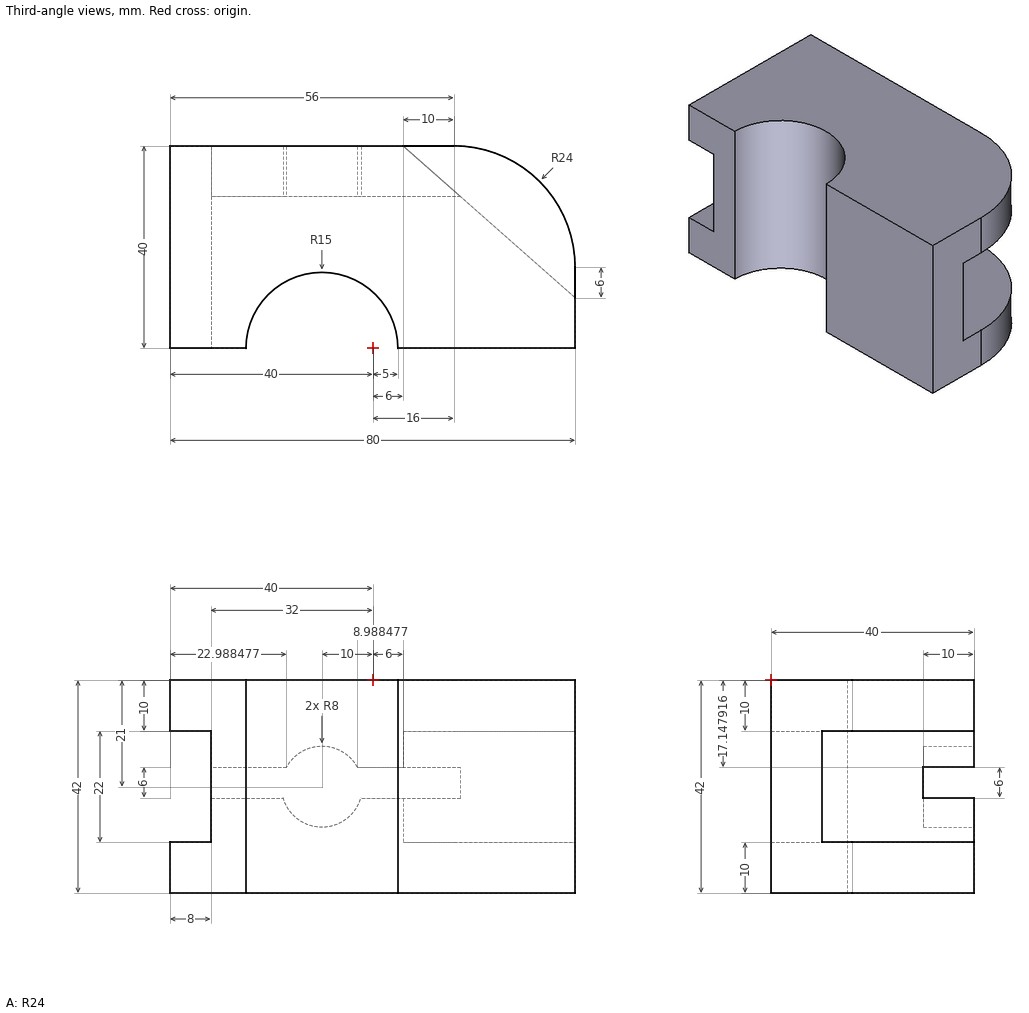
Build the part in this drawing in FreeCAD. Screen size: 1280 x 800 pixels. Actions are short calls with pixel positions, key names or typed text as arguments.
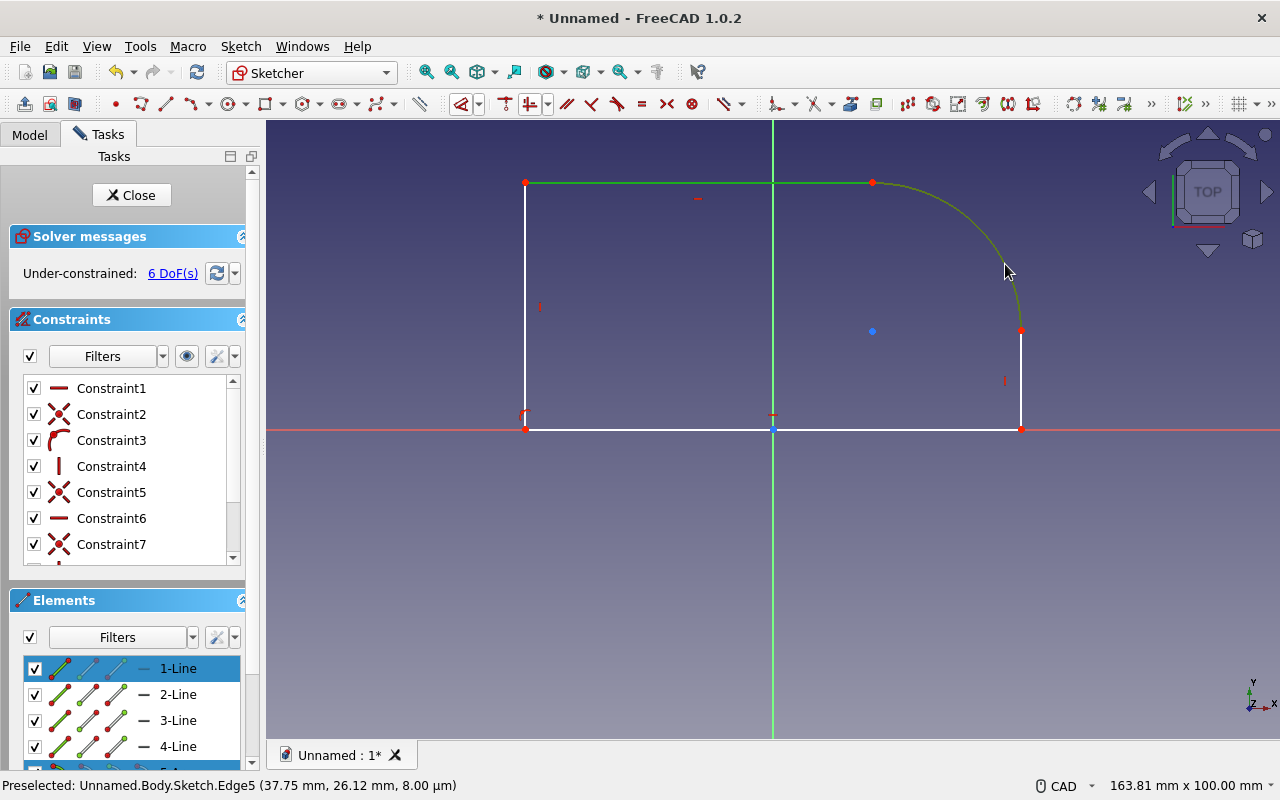
click(617, 104)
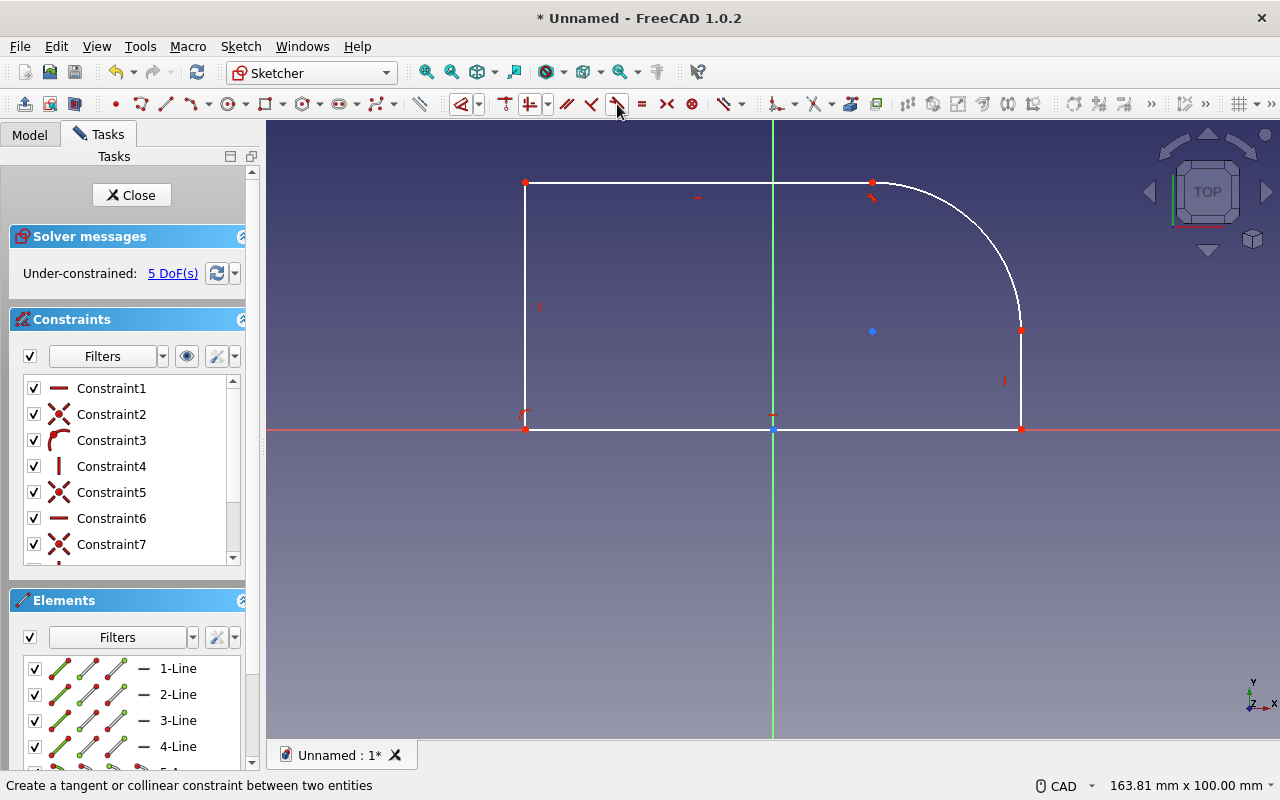
click(1021, 400)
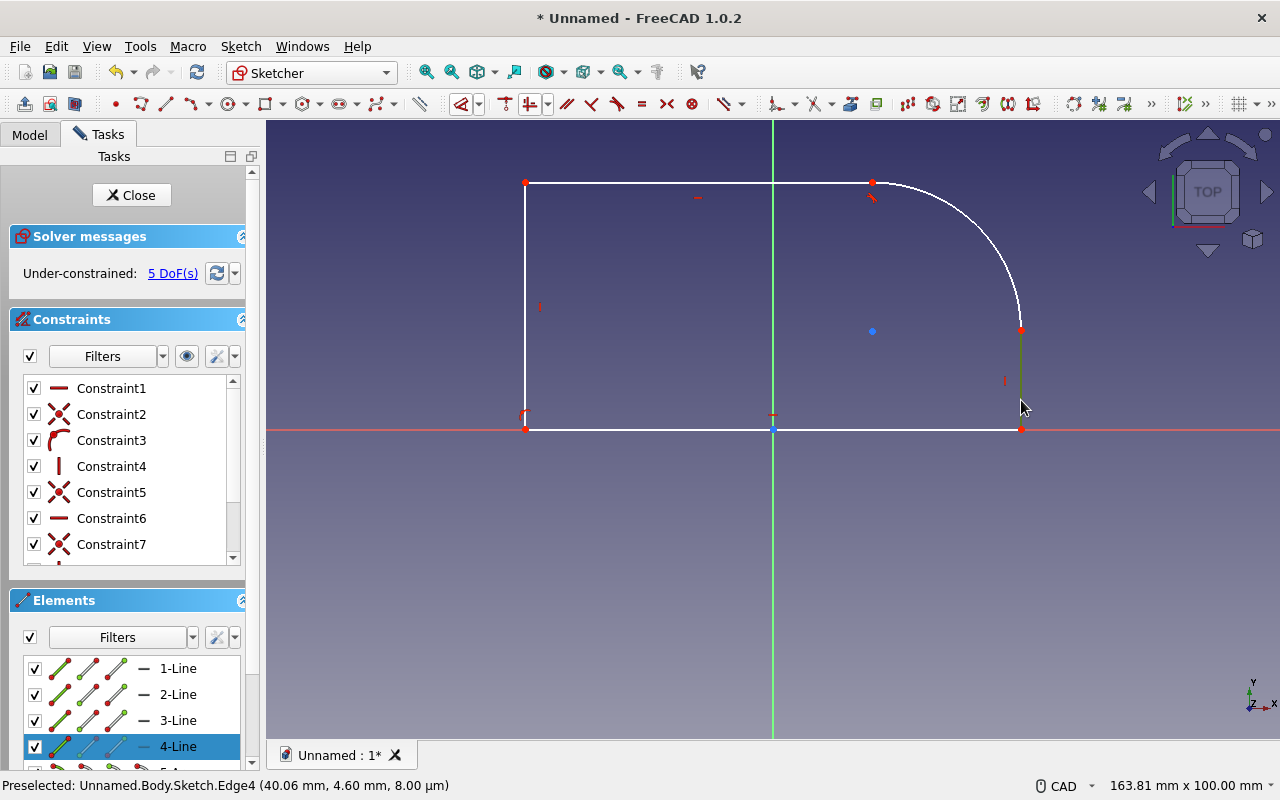
click(1005, 264)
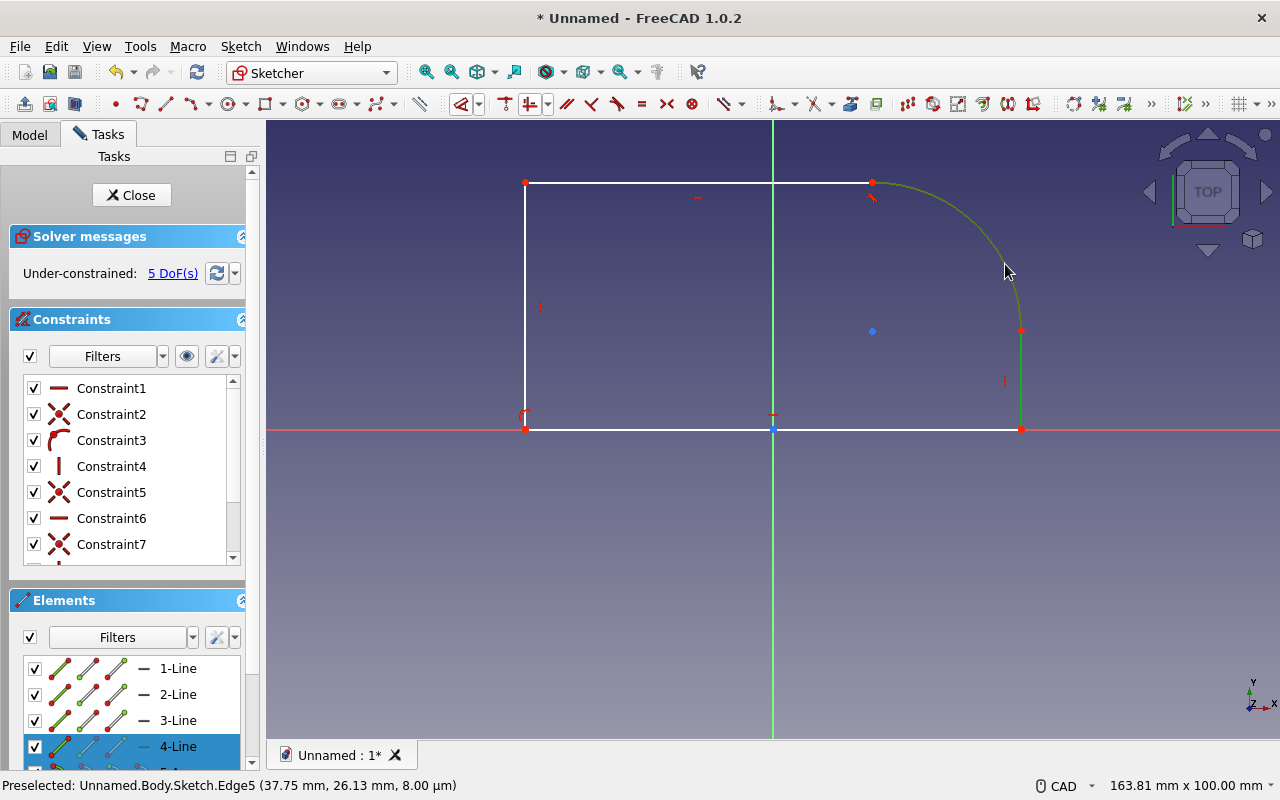
click(617, 104)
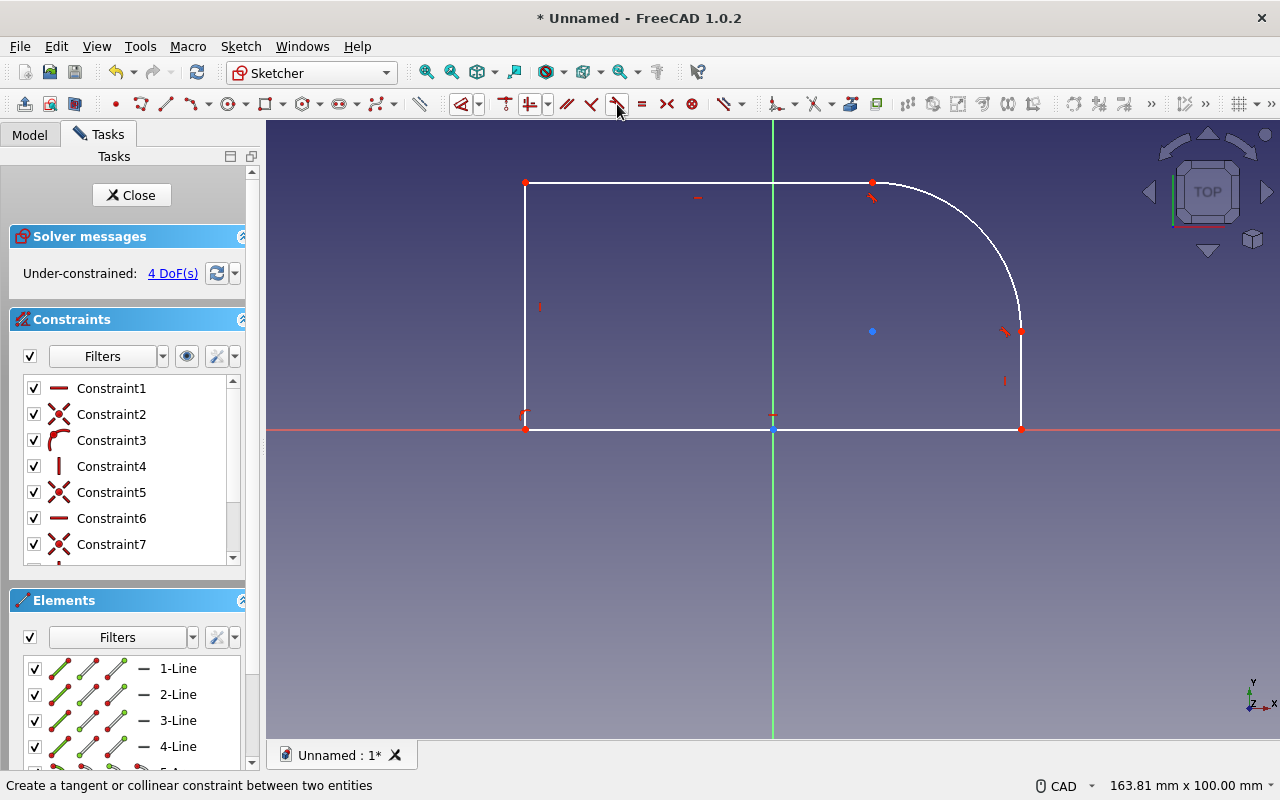
click(460, 104)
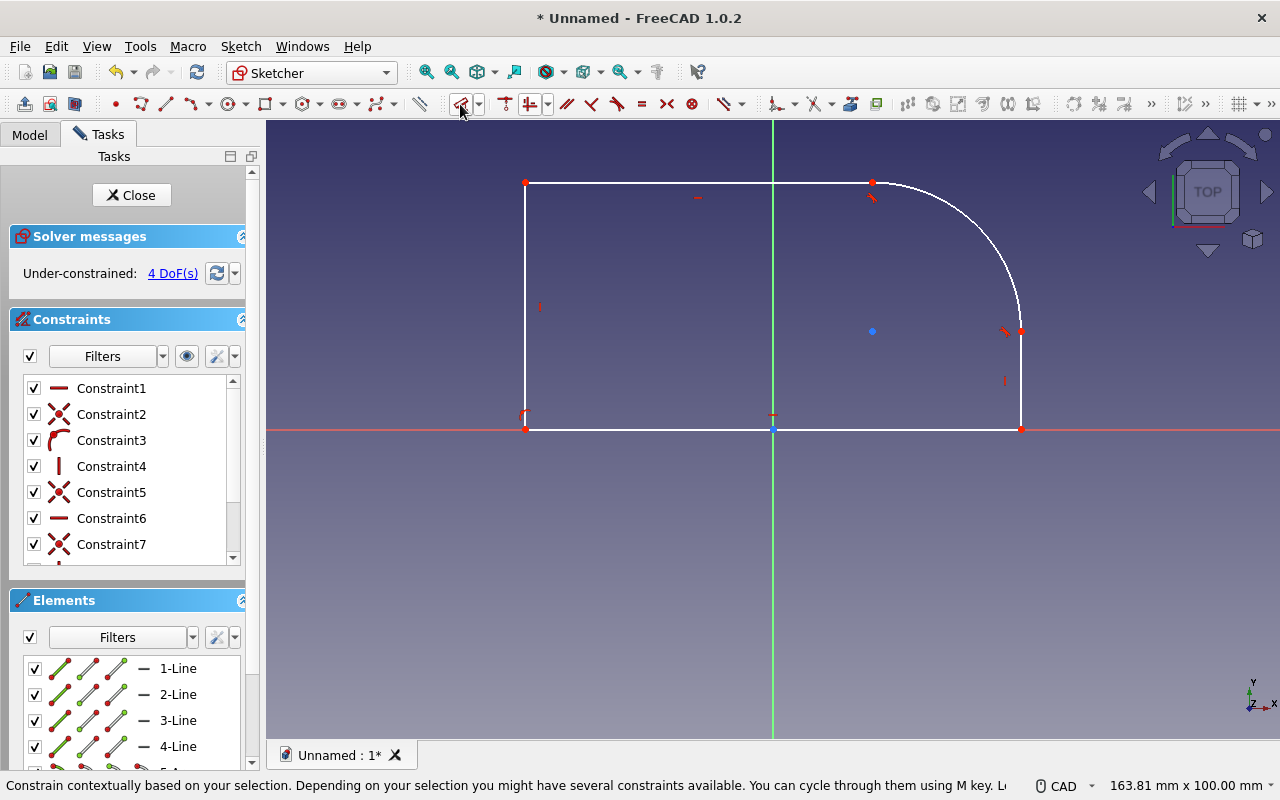
click(1005, 264)
click(1034, 250)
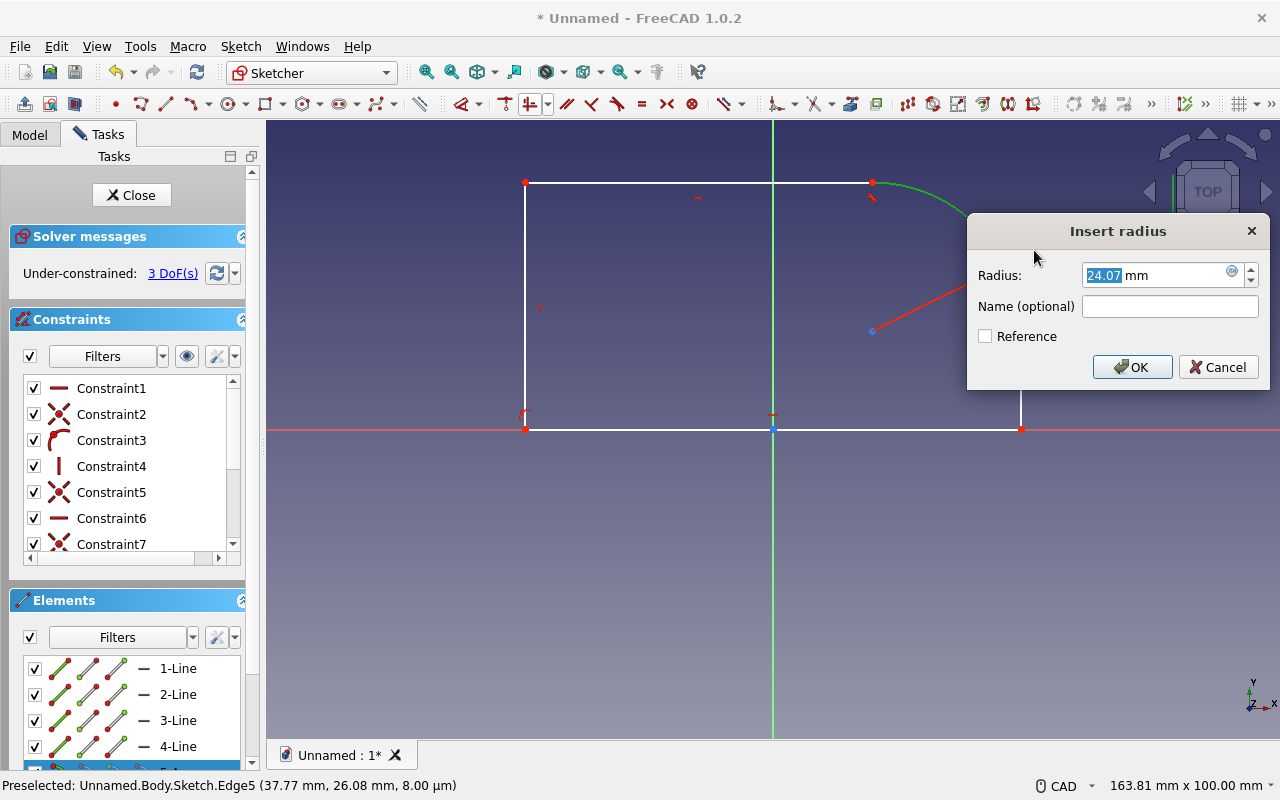
text(24)
key(Return)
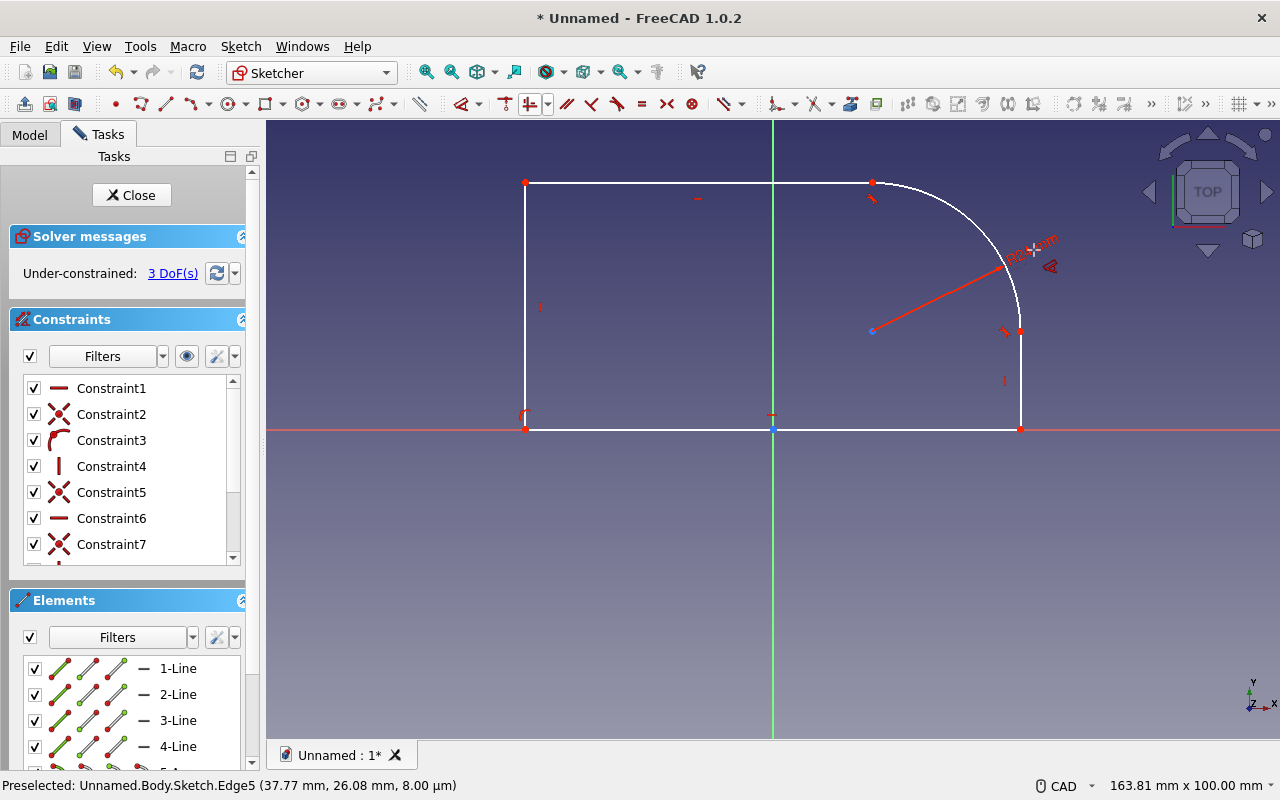
click(629, 183)
click(699, 149)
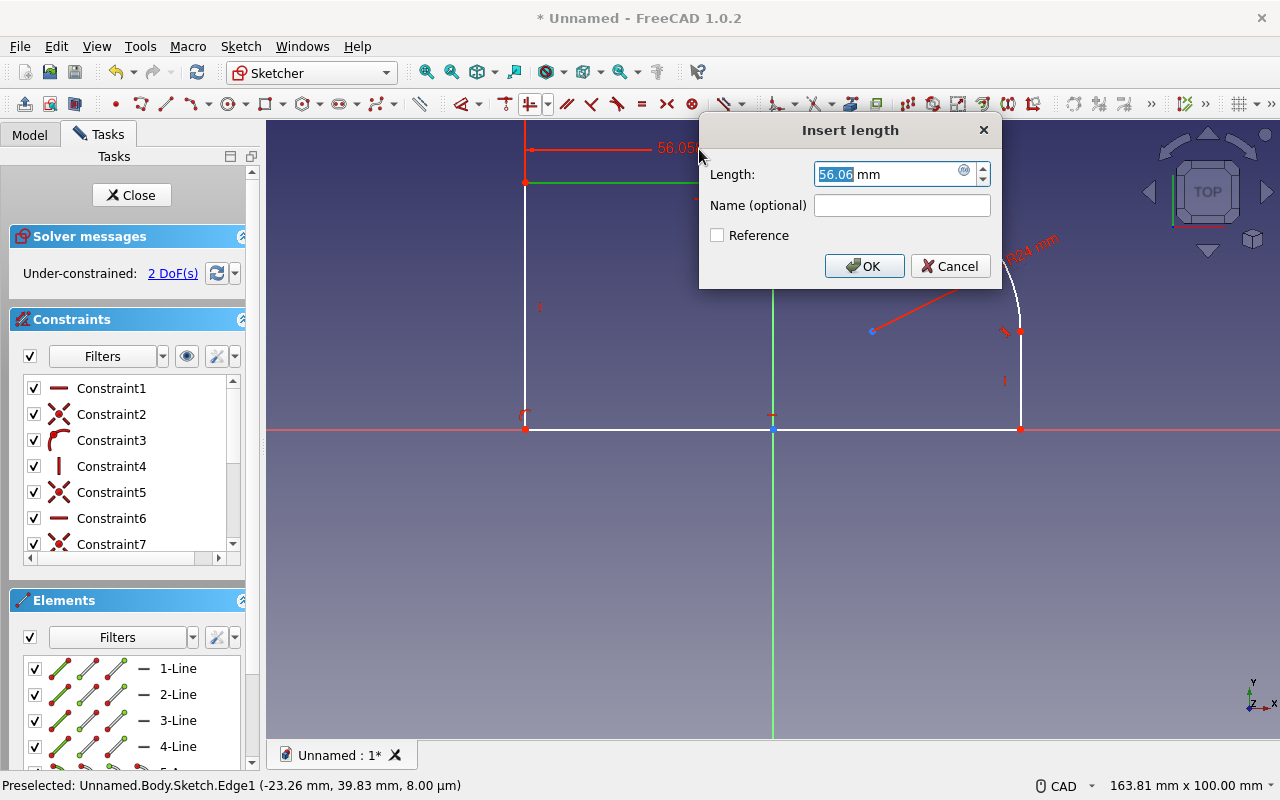
text(56)
key(Return)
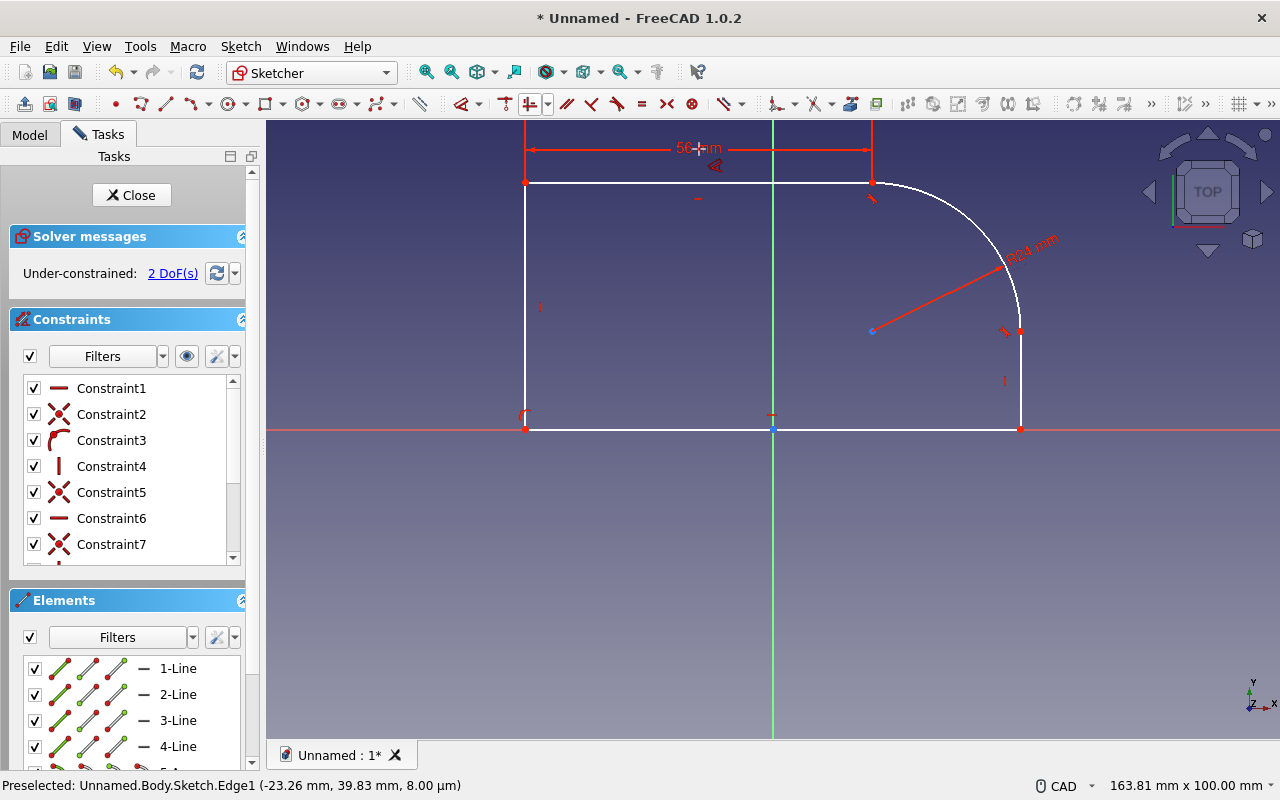
click(525, 257)
click(491, 306)